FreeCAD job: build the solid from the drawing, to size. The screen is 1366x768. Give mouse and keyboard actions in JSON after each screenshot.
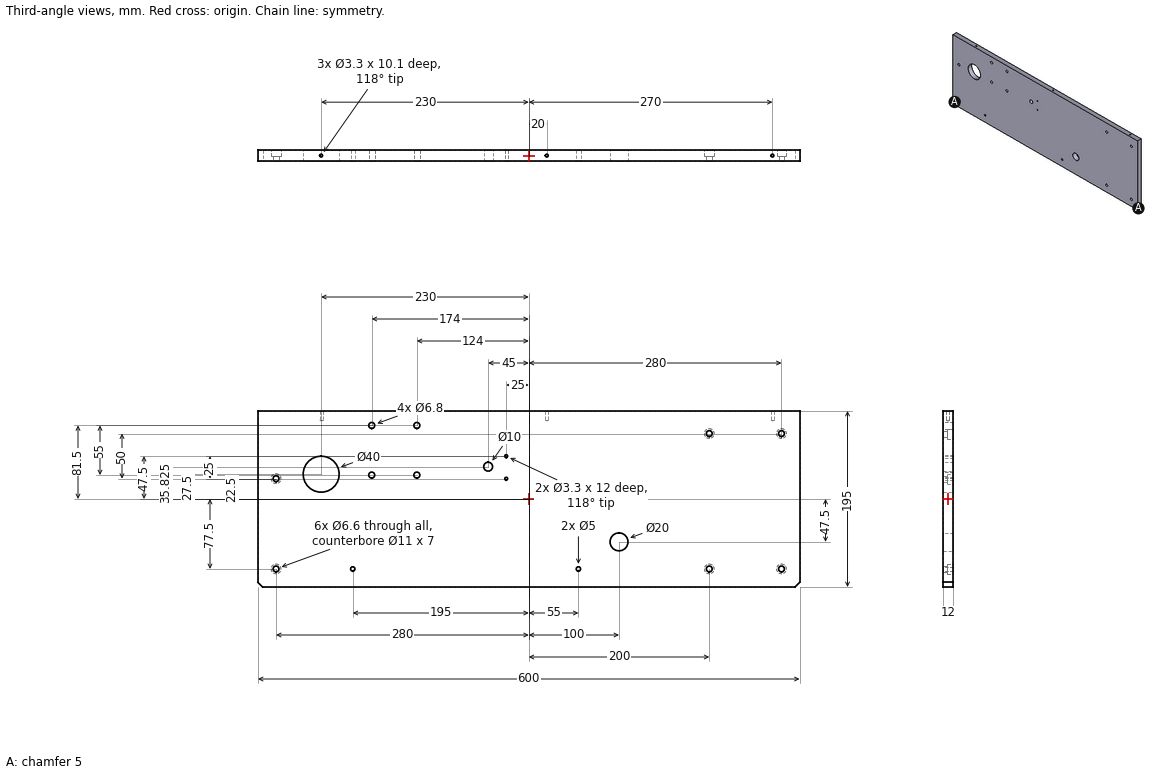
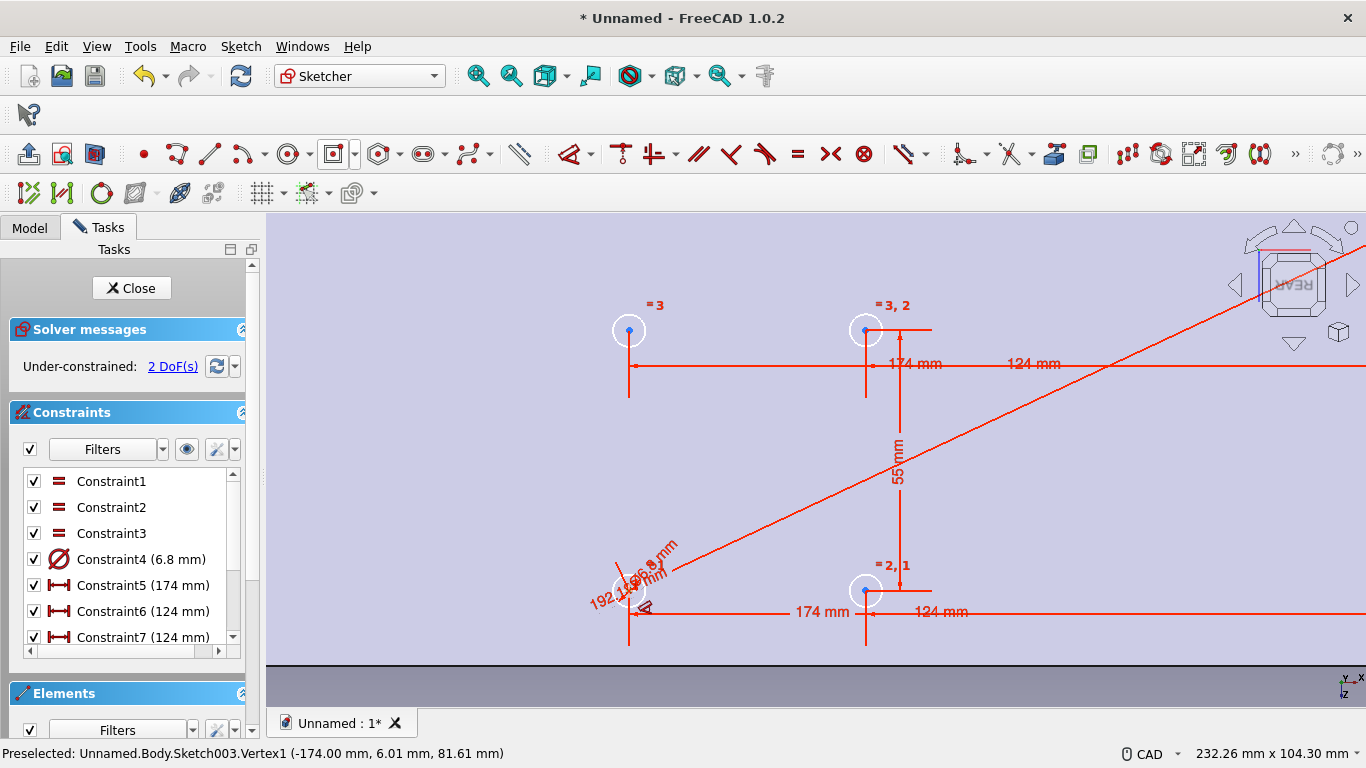
{"action": "left_click", "coordinate": [866, 330]}
{"action": "left_click", "coordinate": [900, 401]}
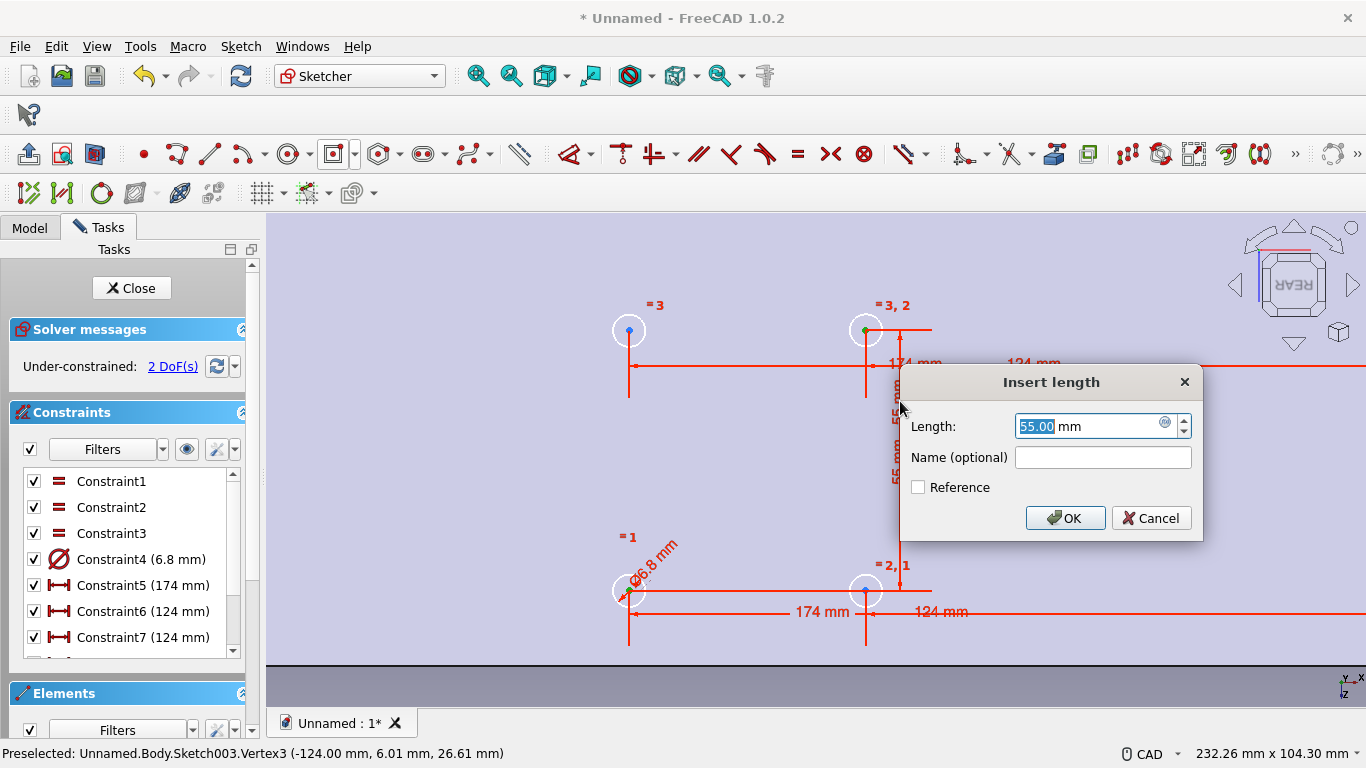
{"action": "type", "text": "55"}
{"action": "key", "text": "Return"}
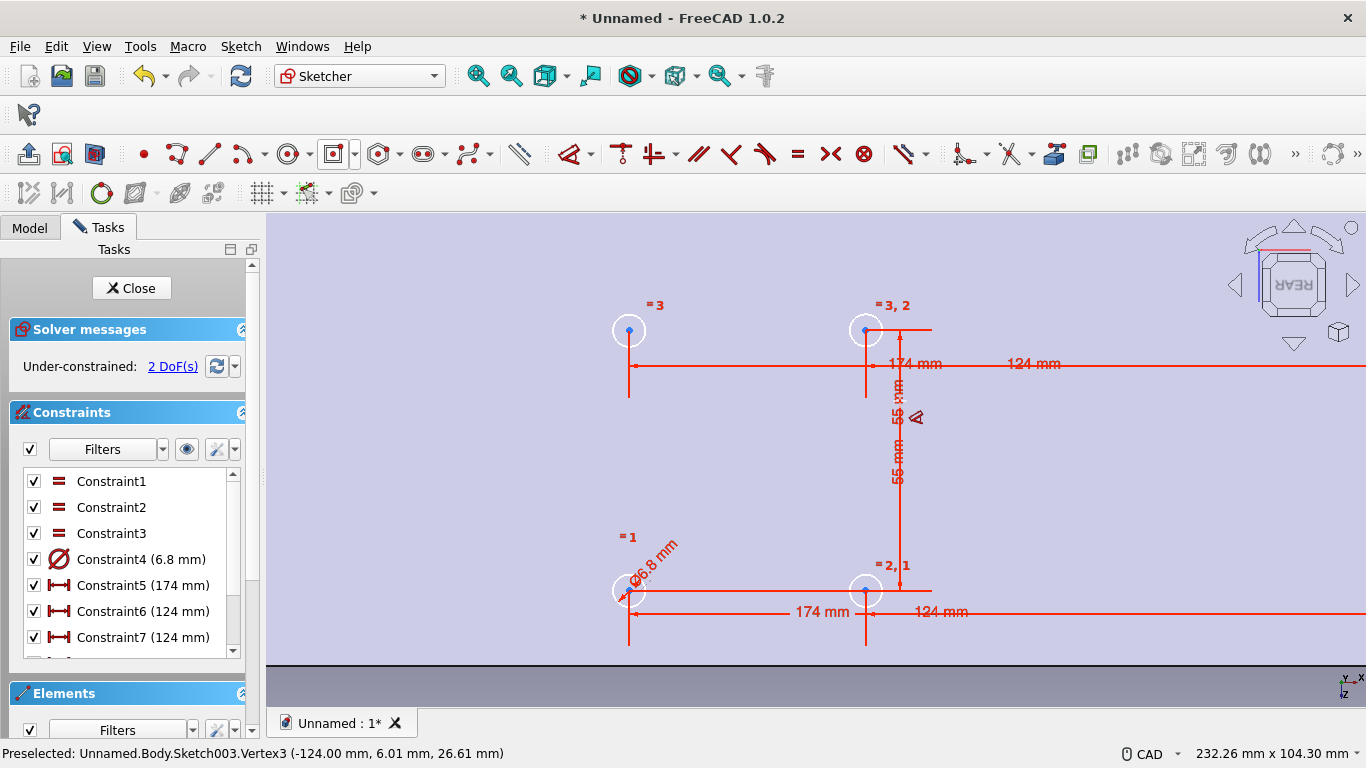
{"action": "left_click", "coordinate": [629, 591]}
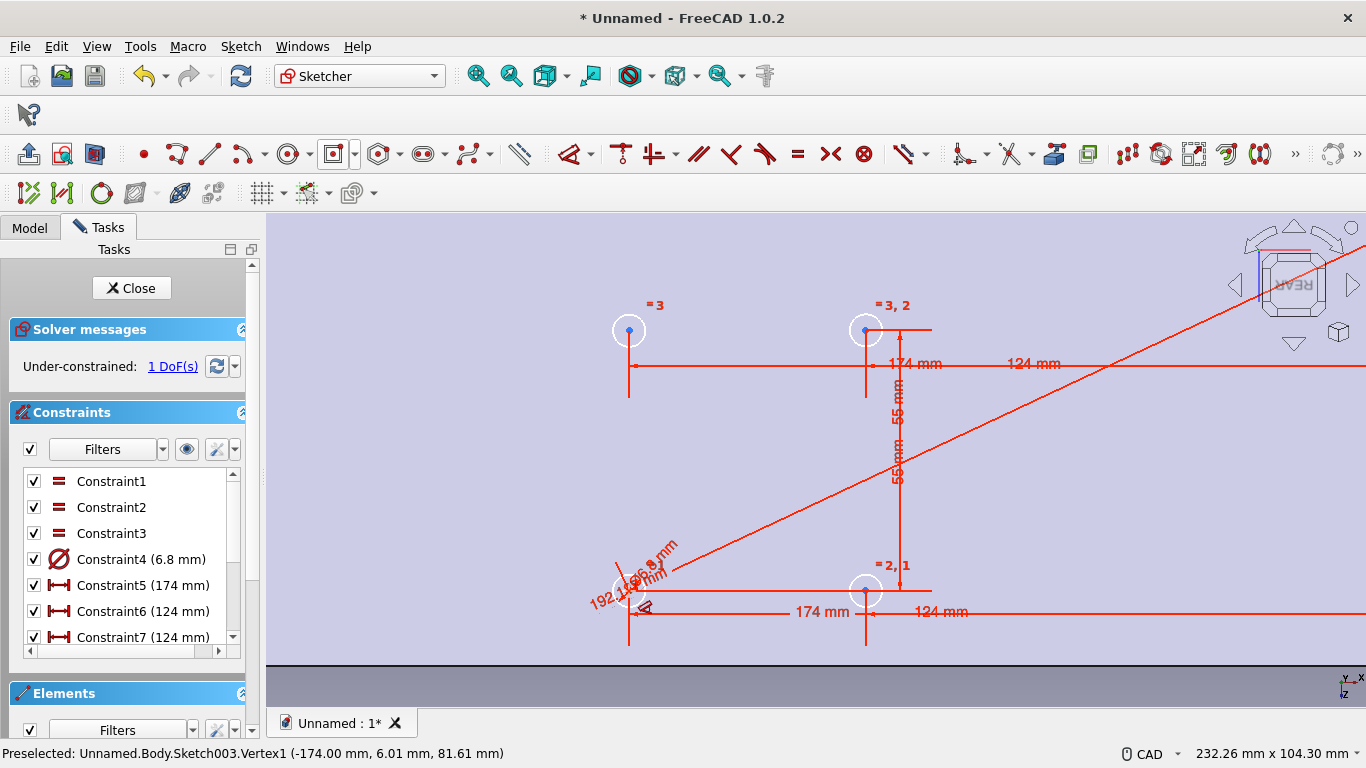
{"action": "left_click", "coordinate": [629, 331]}
{"action": "left_click", "coordinate": [595, 461]}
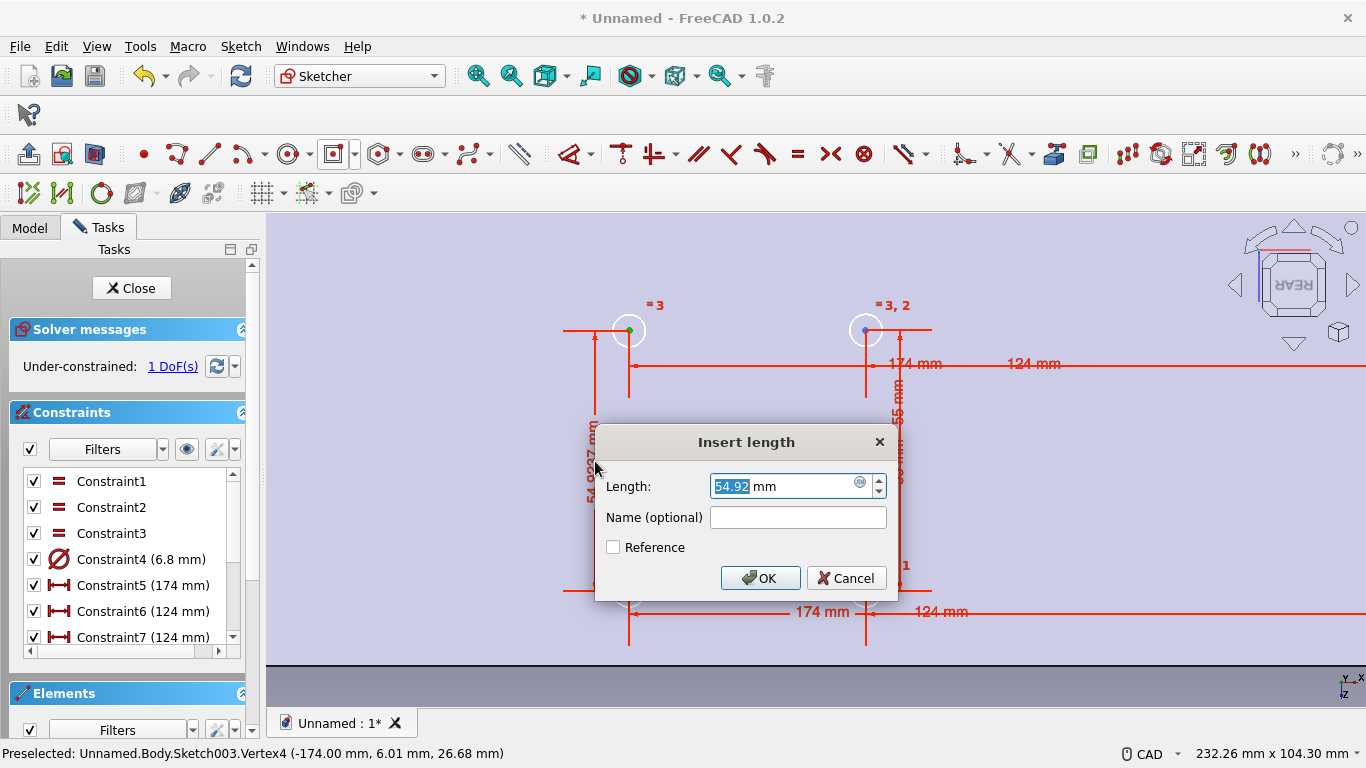
{"action": "type", "text": "55"}
{"action": "key", "text": "Return"}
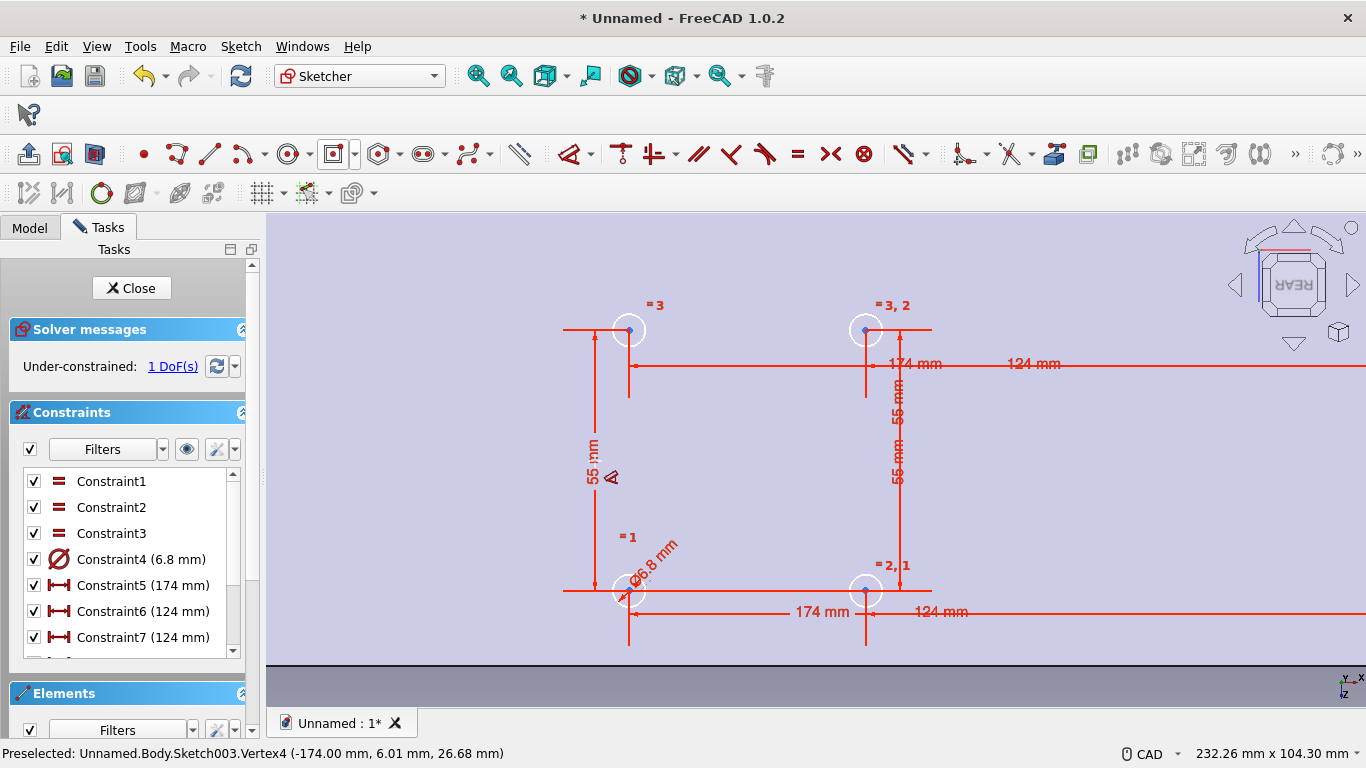
{"action": "left_click", "coordinate": [629, 591]}
{"action": "left_click", "coordinate": [595, 416]}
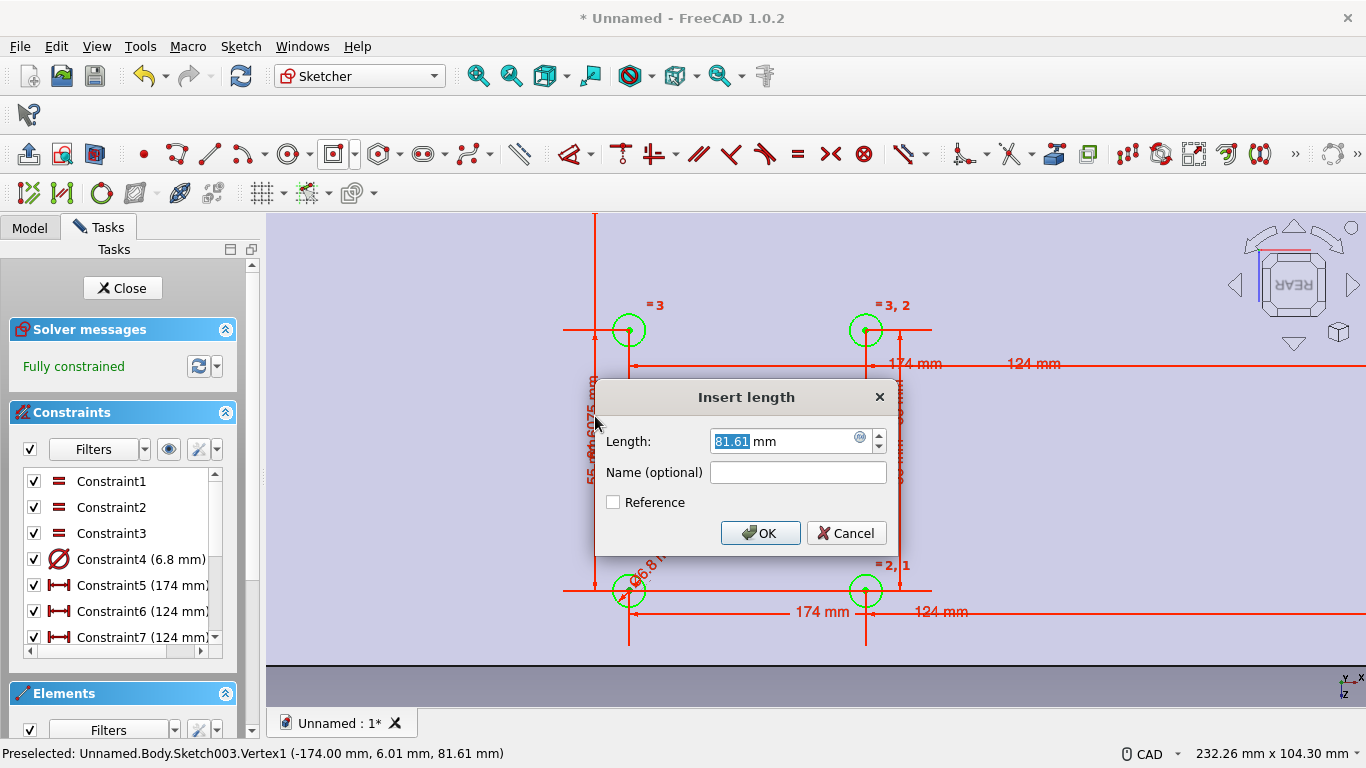
{"action": "type", "text": "81.5"}
{"action": "key", "text": "Return"}
{"action": "key", "text": "Escape"}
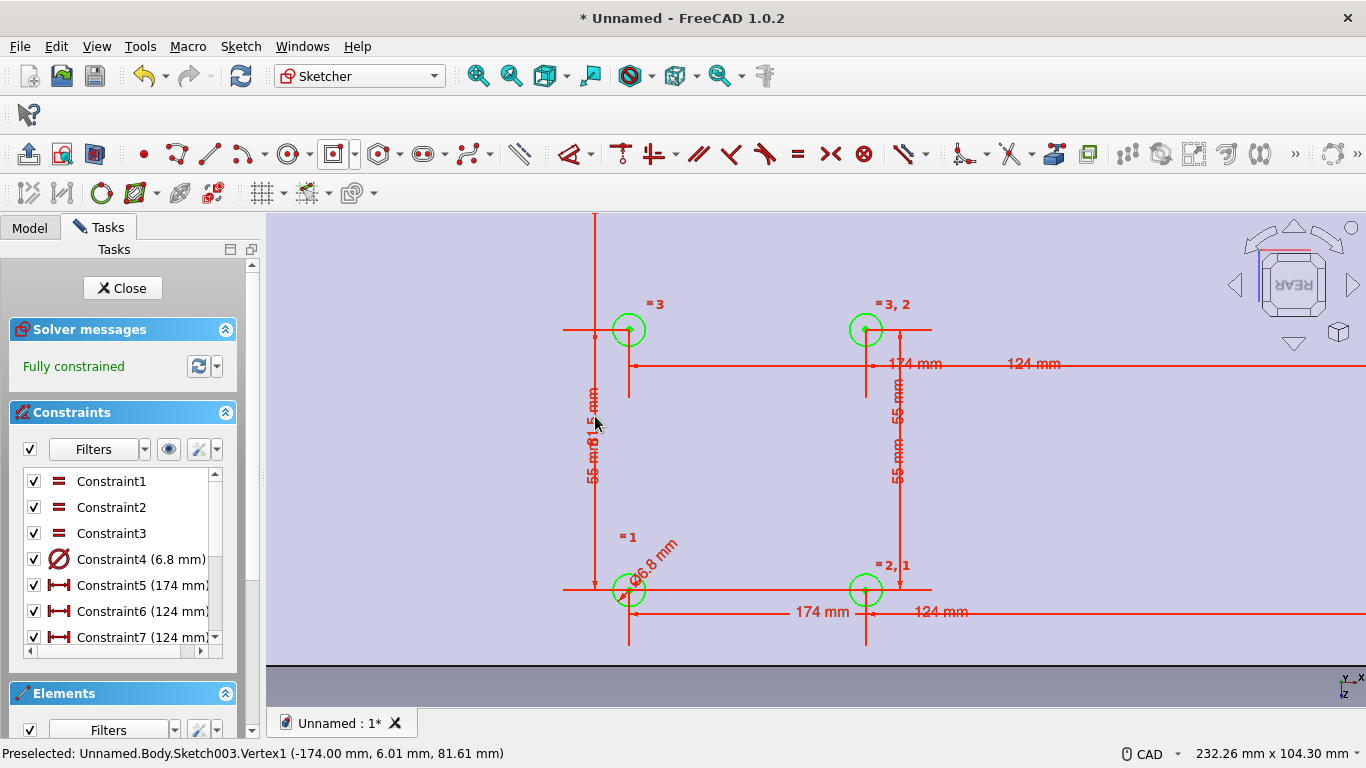
{"action": "left_click", "coordinate": [123, 288]}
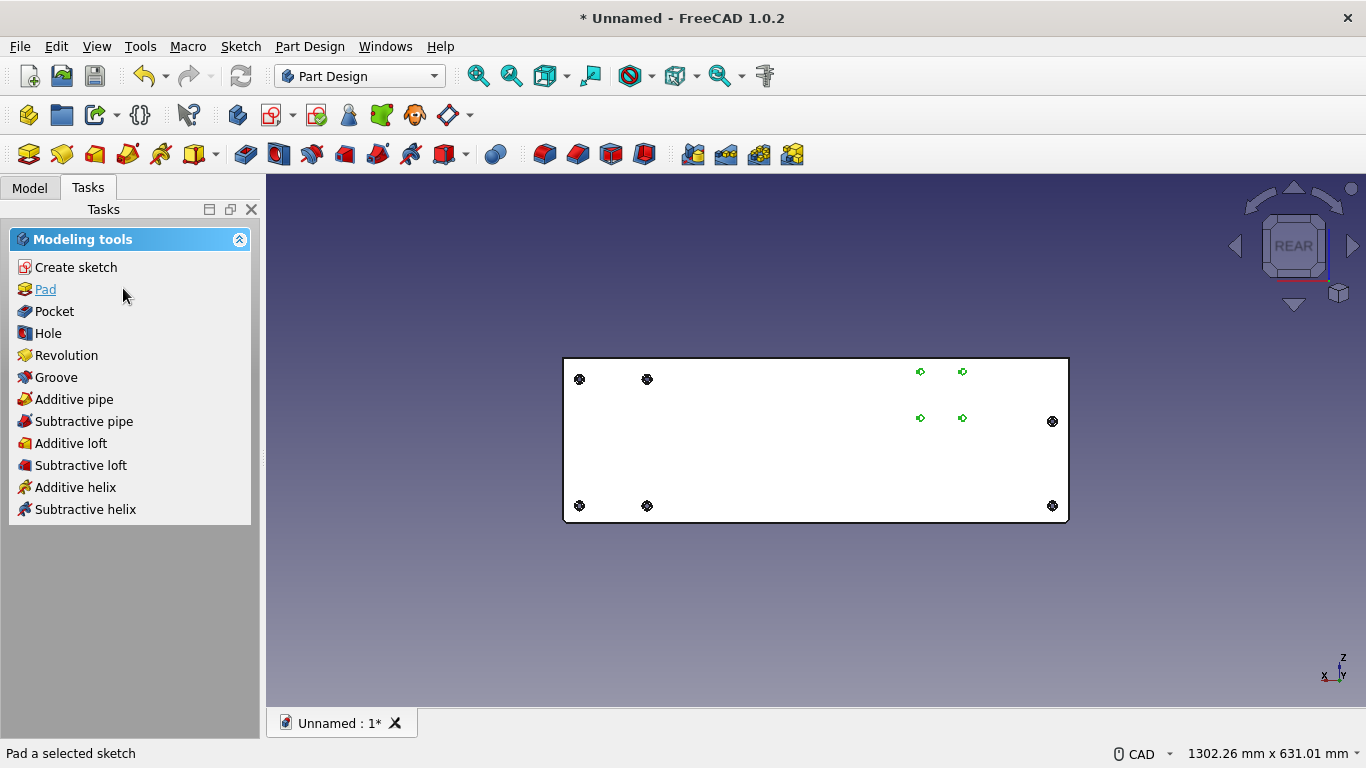
{"action": "left_click", "coordinate": [246, 154]}